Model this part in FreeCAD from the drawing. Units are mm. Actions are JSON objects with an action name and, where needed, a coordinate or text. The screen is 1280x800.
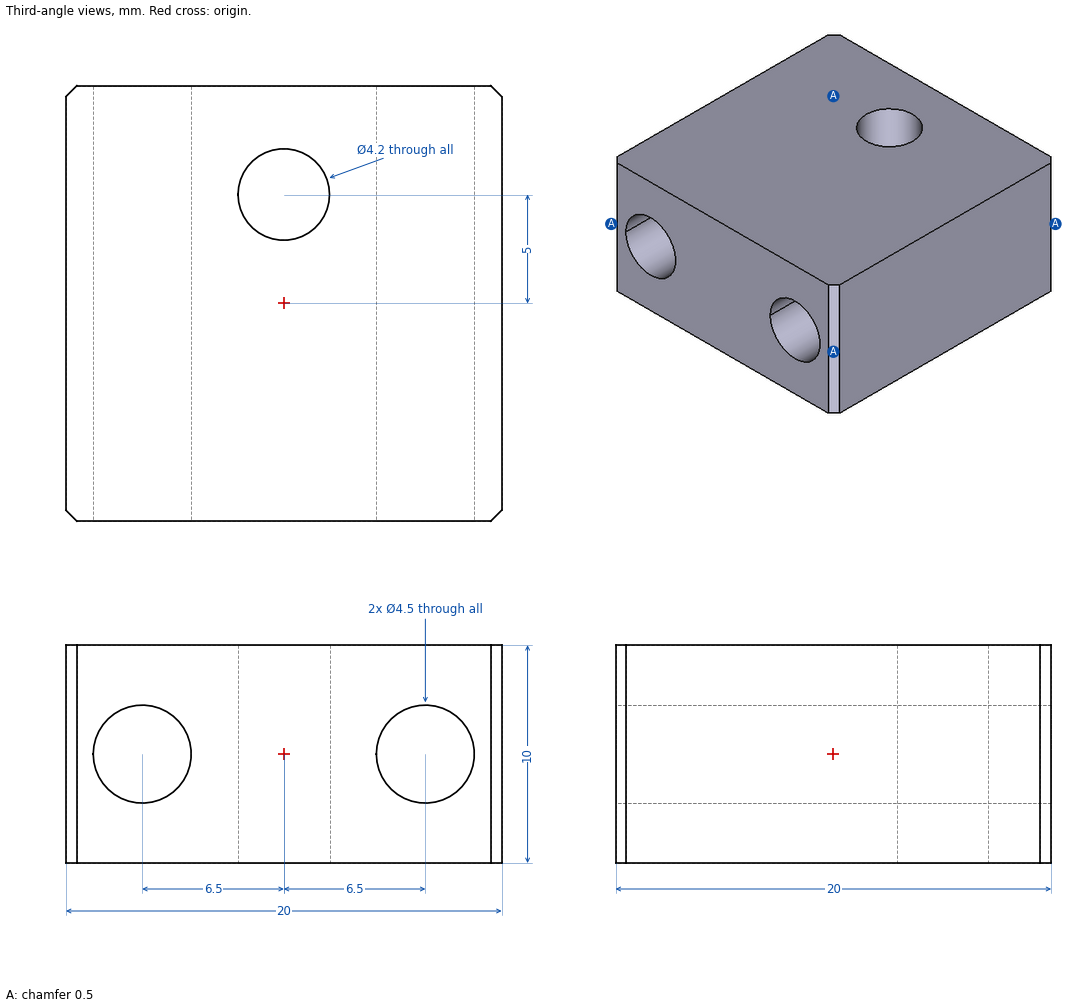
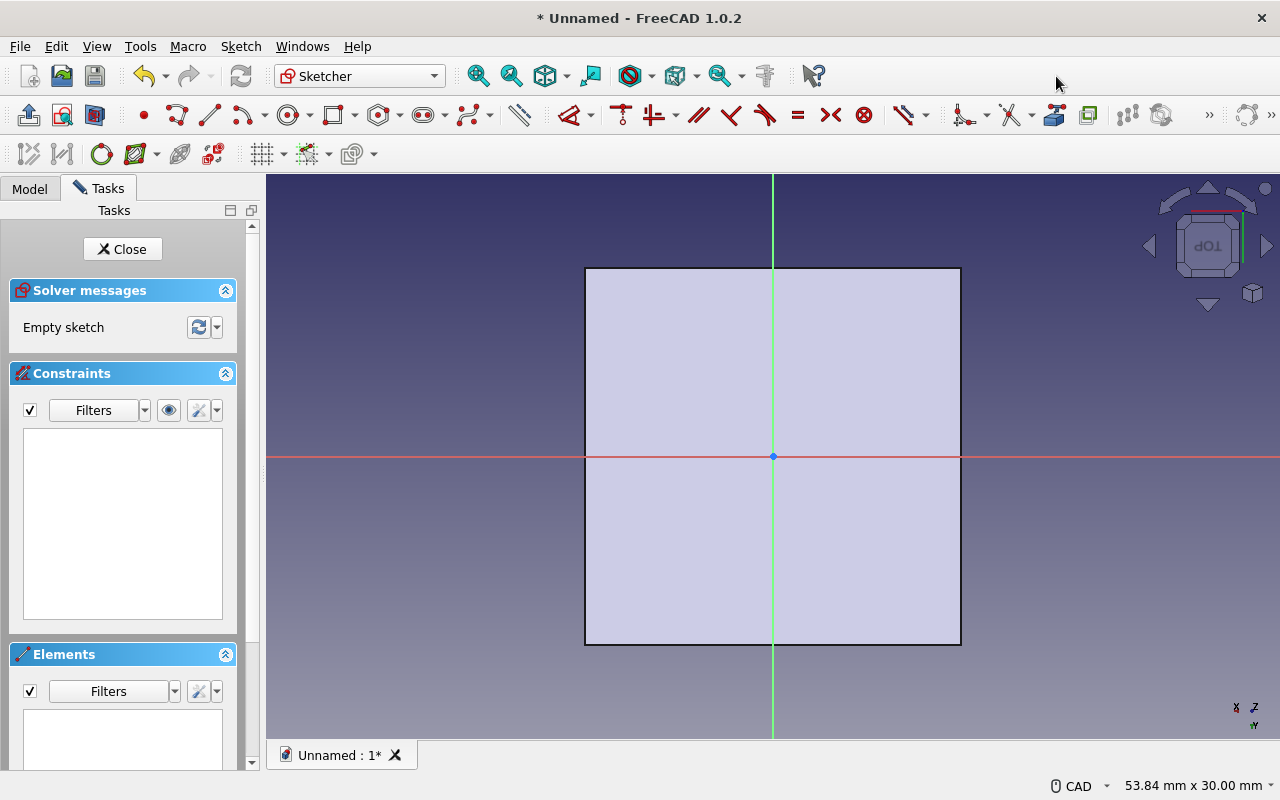
{"action": "scroll", "coordinate": [813, 562], "scroll_direction": "up", "scroll_amount": 5}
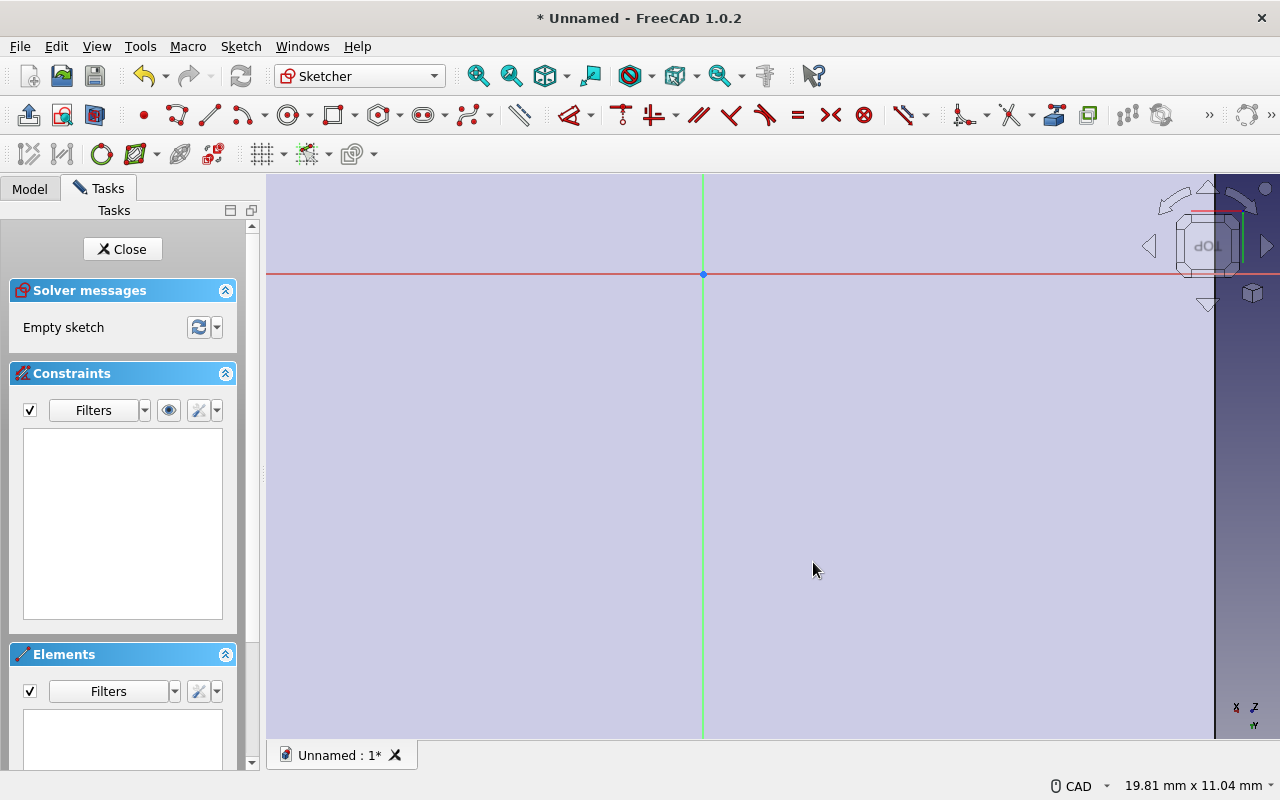
{"action": "left_click", "coordinate": [288, 116]}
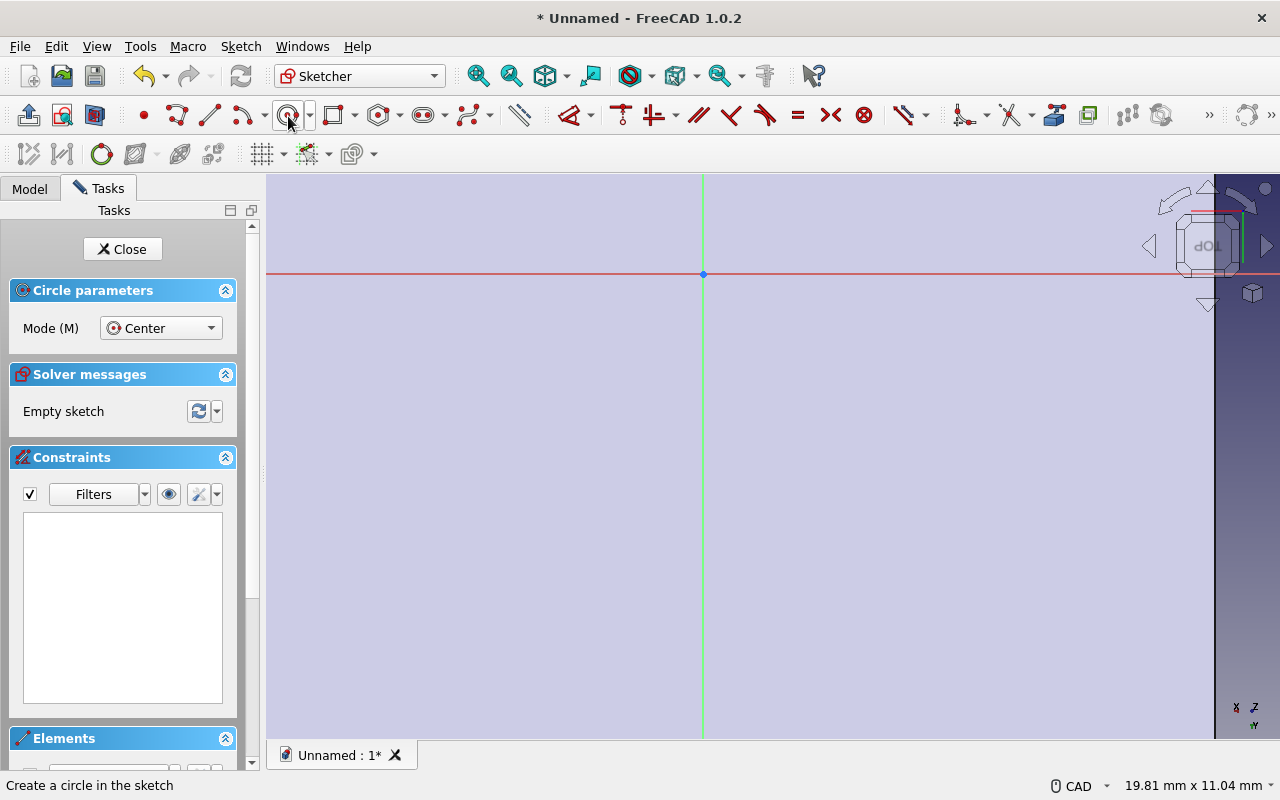
{"action": "left_click", "coordinate": [703, 530]}
{"action": "left_click", "coordinate": [779, 454]}
{"action": "key", "text": "Escape"}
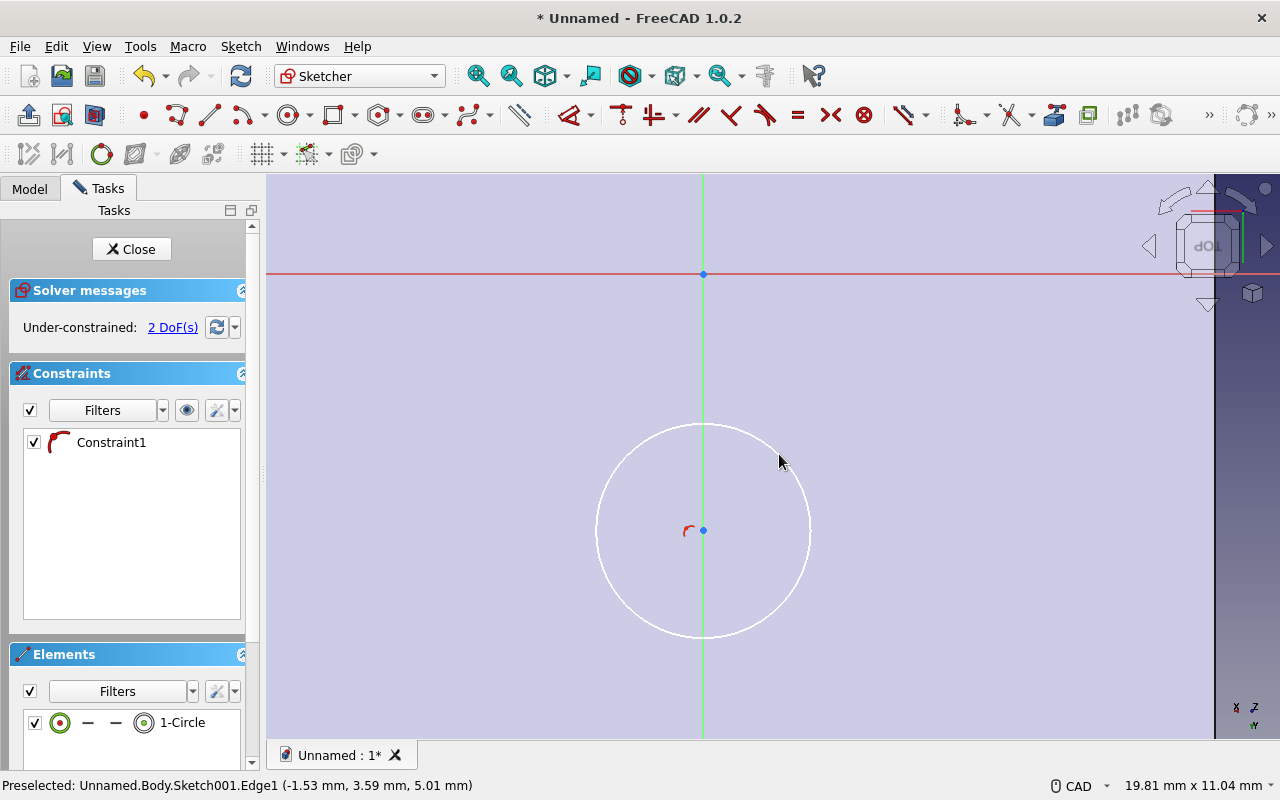
{"action": "key", "text": "d"}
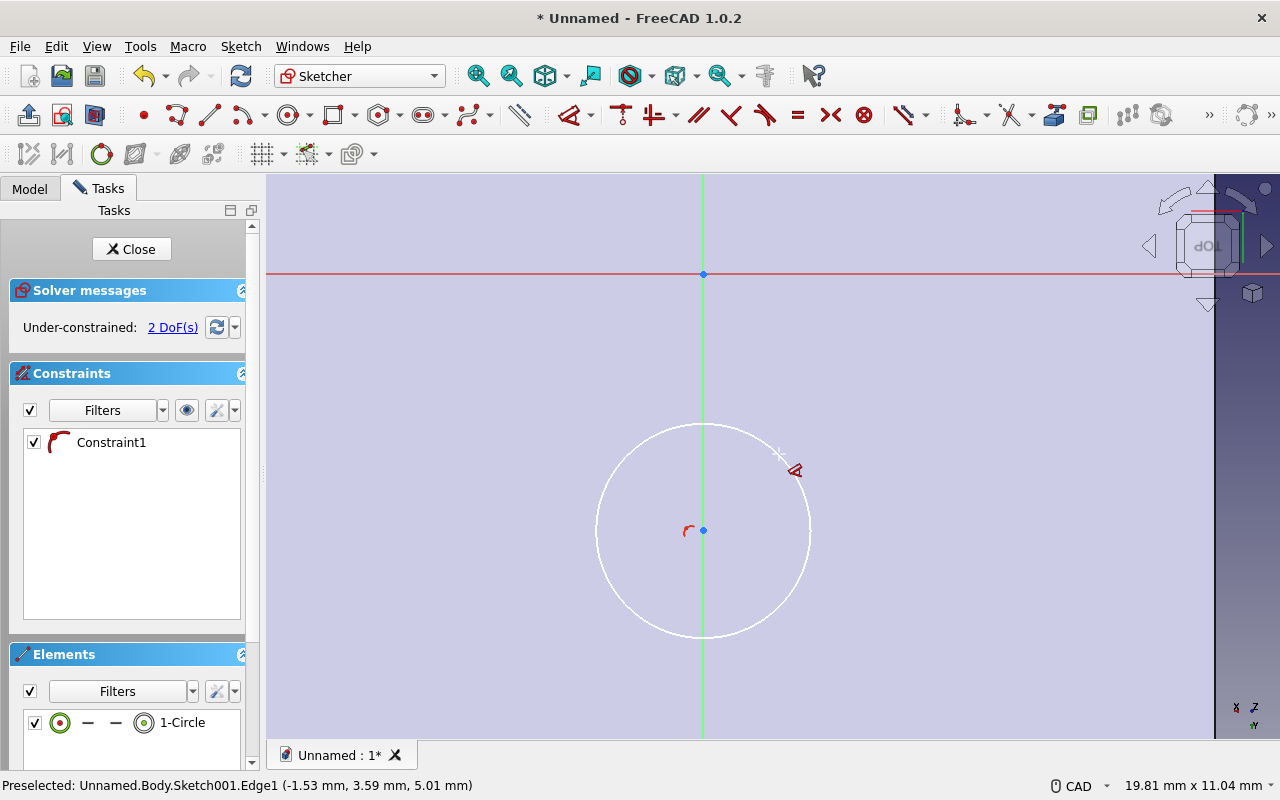
{"action": "left_click", "coordinate": [779, 455]}
{"action": "left_click", "coordinate": [802, 432]}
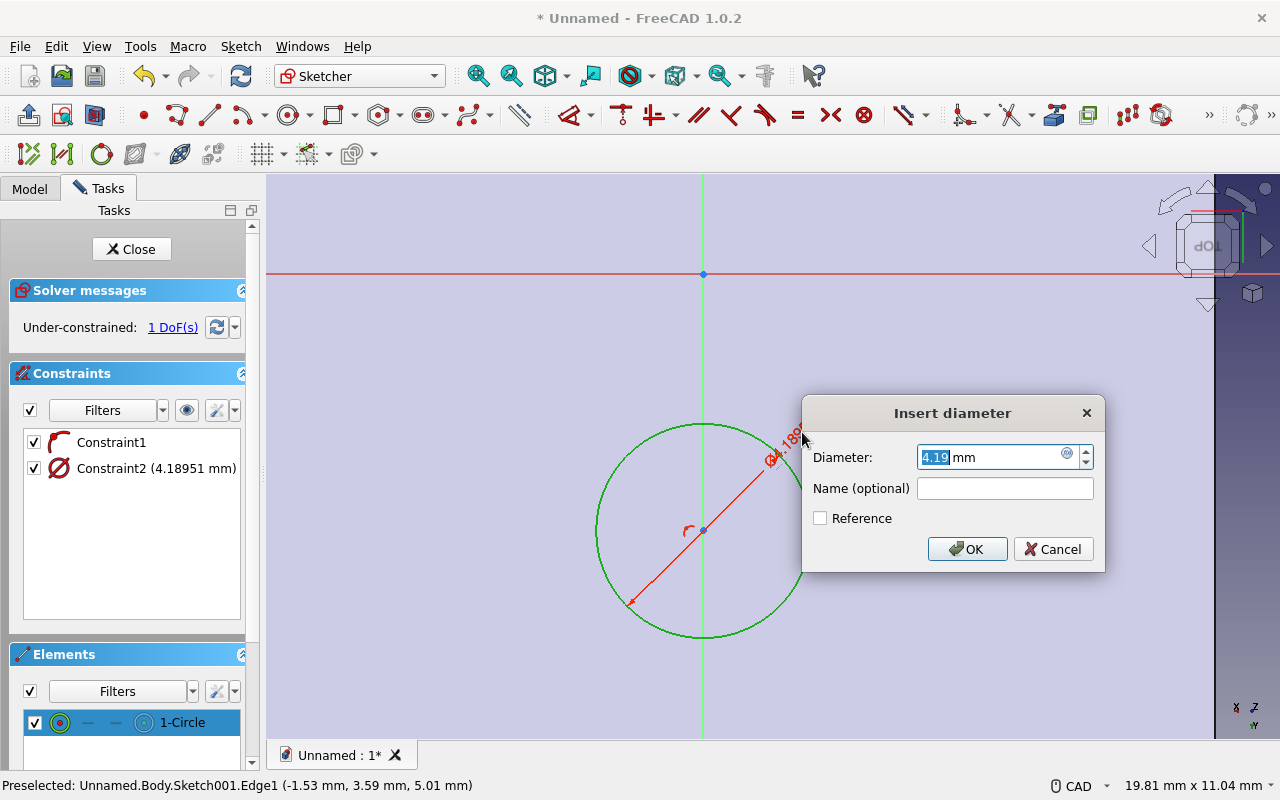
{"action": "type", "text": "4.2"}
{"action": "key", "text": "Return"}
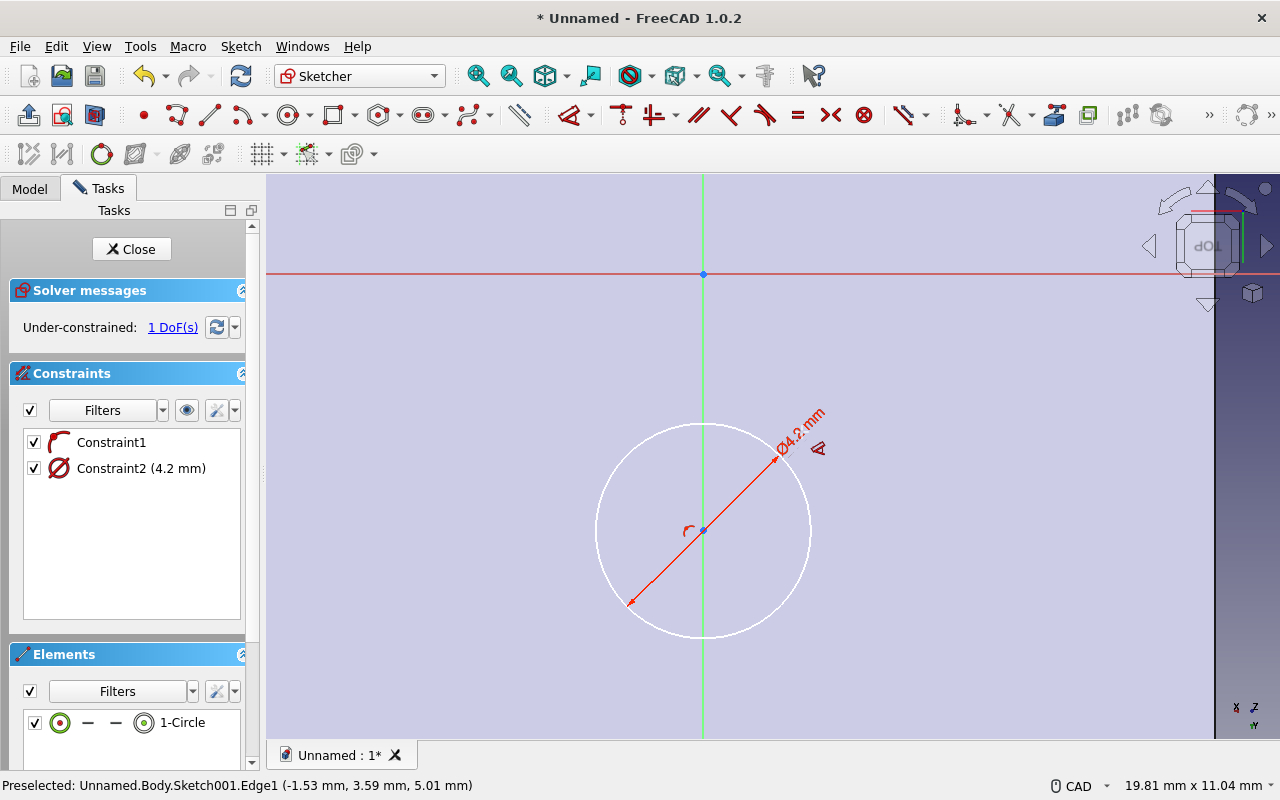
{"action": "left_click", "coordinate": [703, 531]}
{"action": "left_click", "coordinate": [737, 403]}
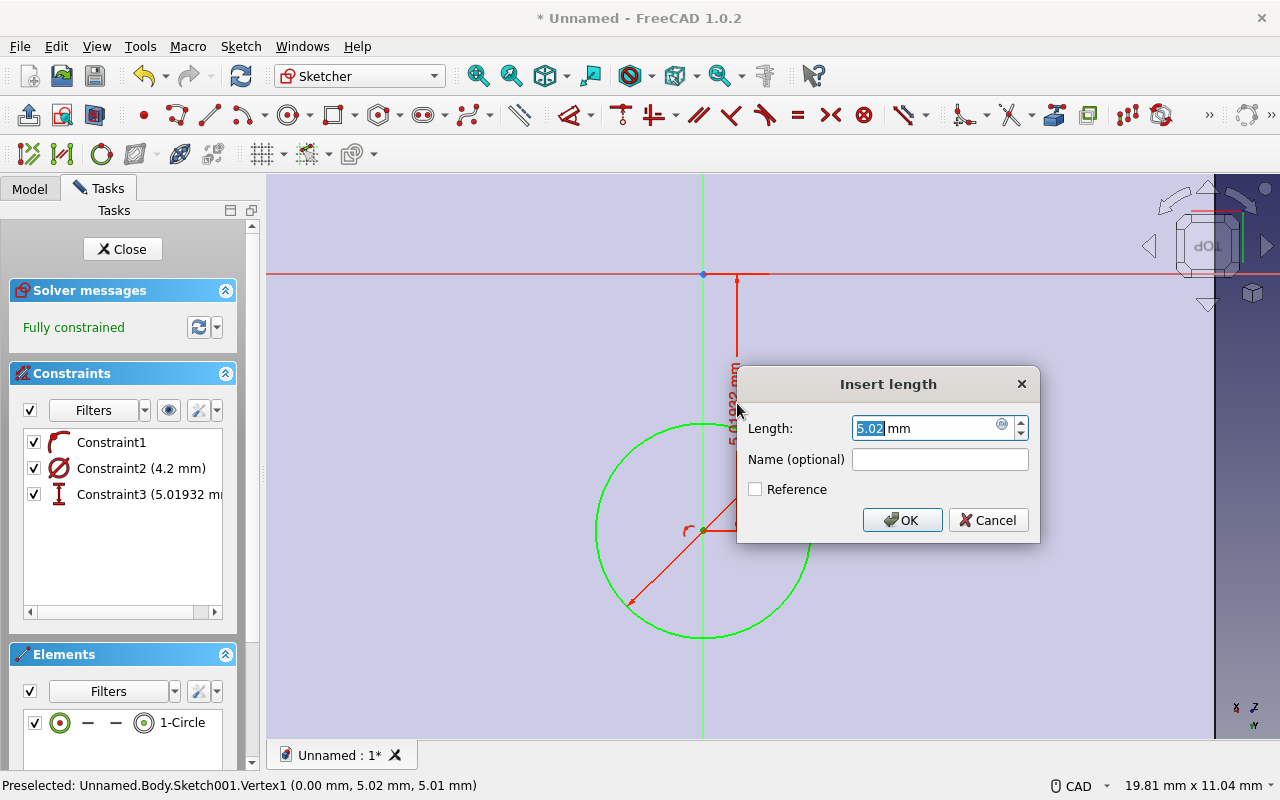
{"action": "type", "text": "5"}
{"action": "key", "text": "Return"}
{"action": "key", "text": "Escape"}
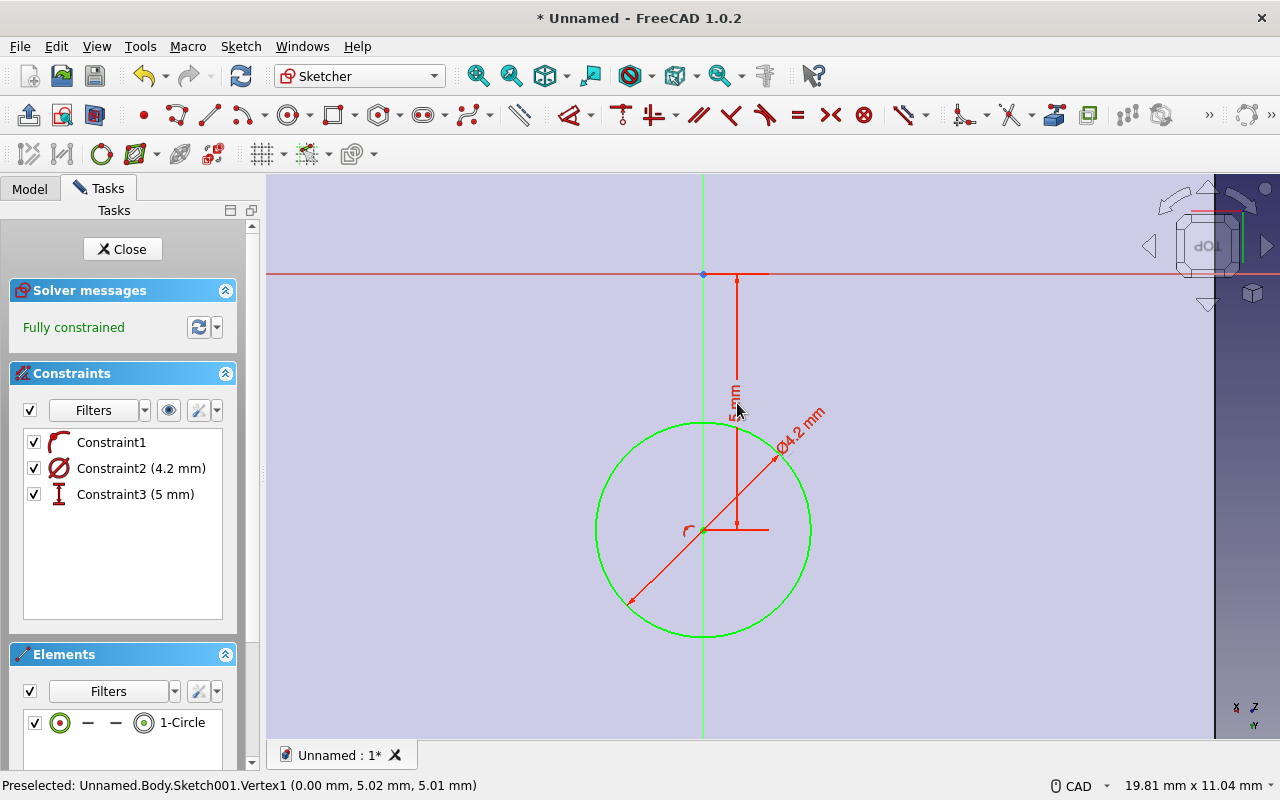
{"action": "left_click", "coordinate": [123, 249]}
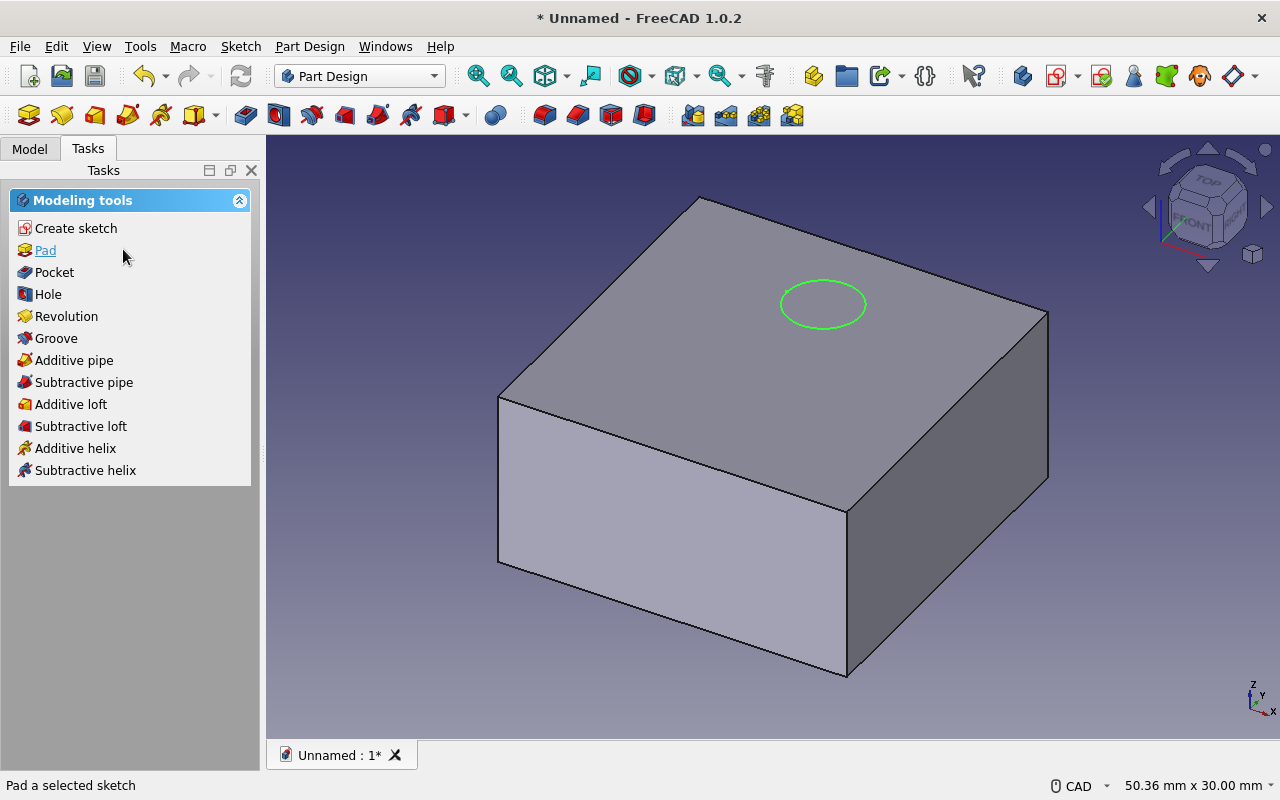
{"action": "left_click", "coordinate": [279, 116]}